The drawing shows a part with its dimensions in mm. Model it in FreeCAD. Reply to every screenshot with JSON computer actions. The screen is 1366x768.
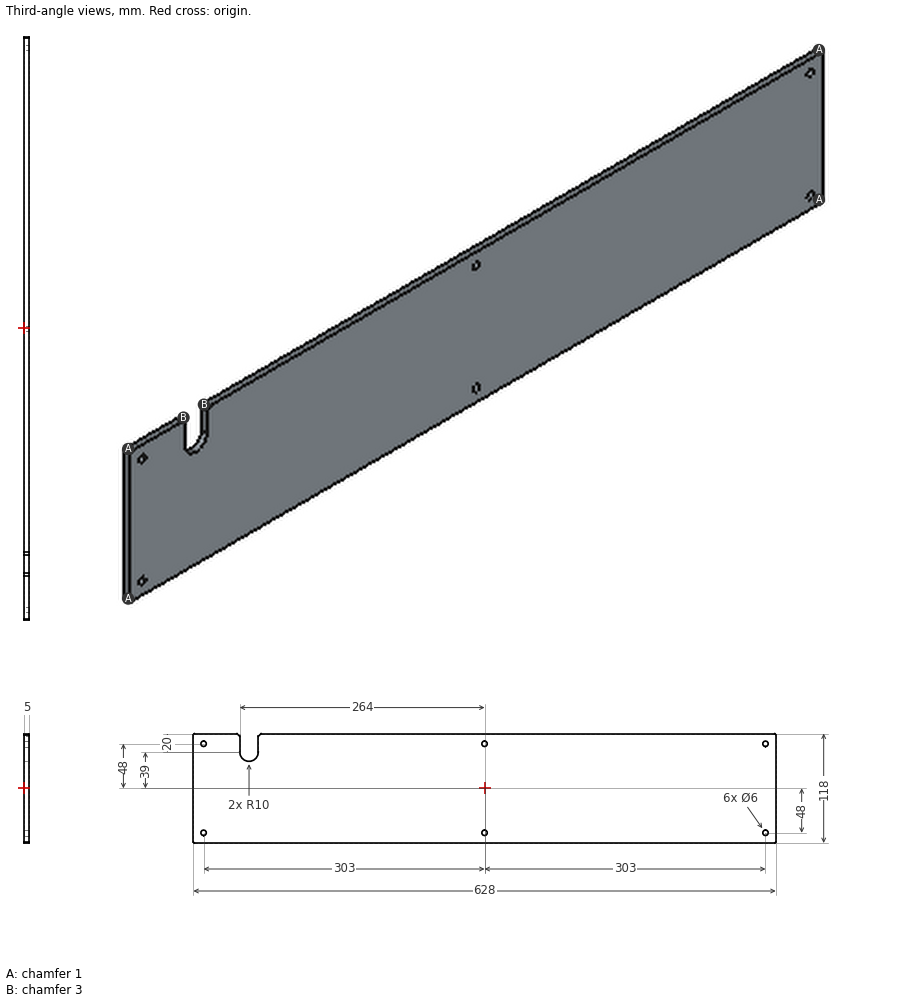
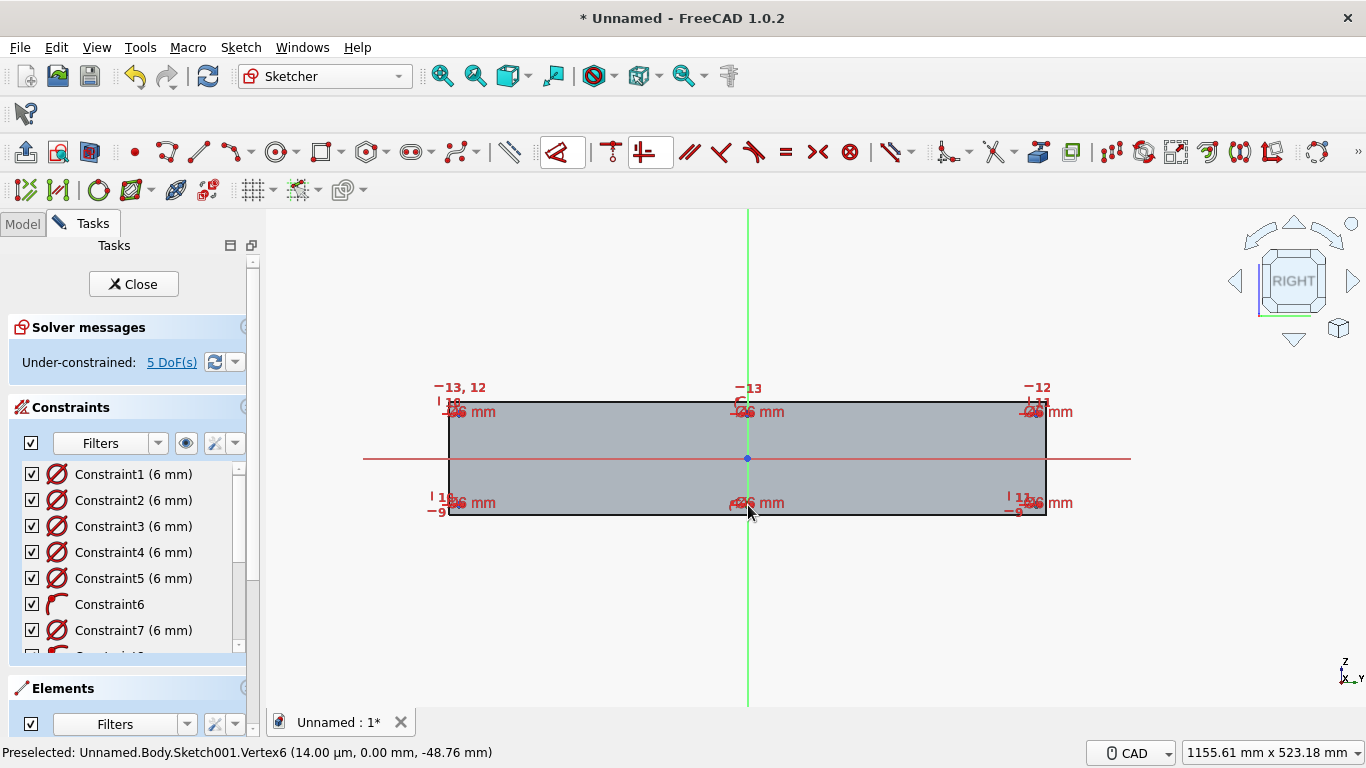
{"action": "key", "text": "h"}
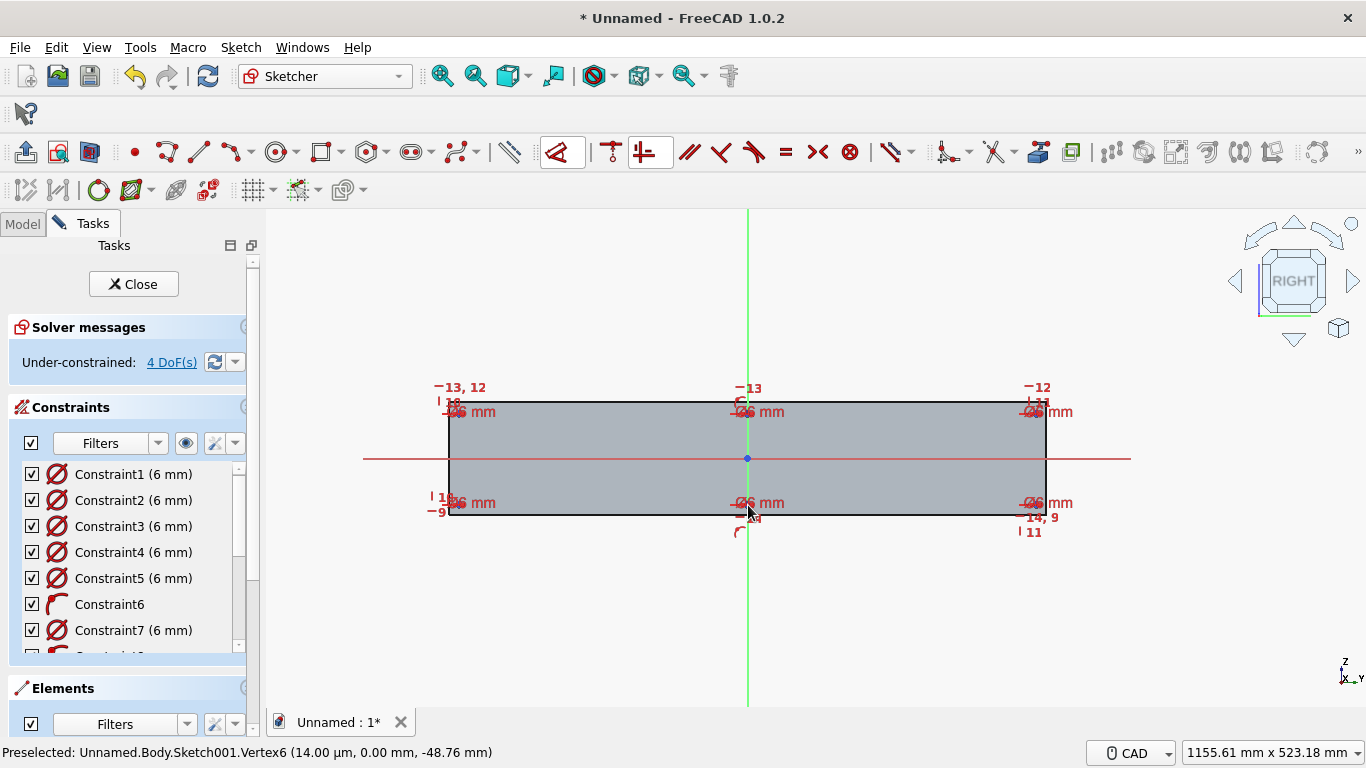
{"action": "left_click", "coordinate": [1036, 505]}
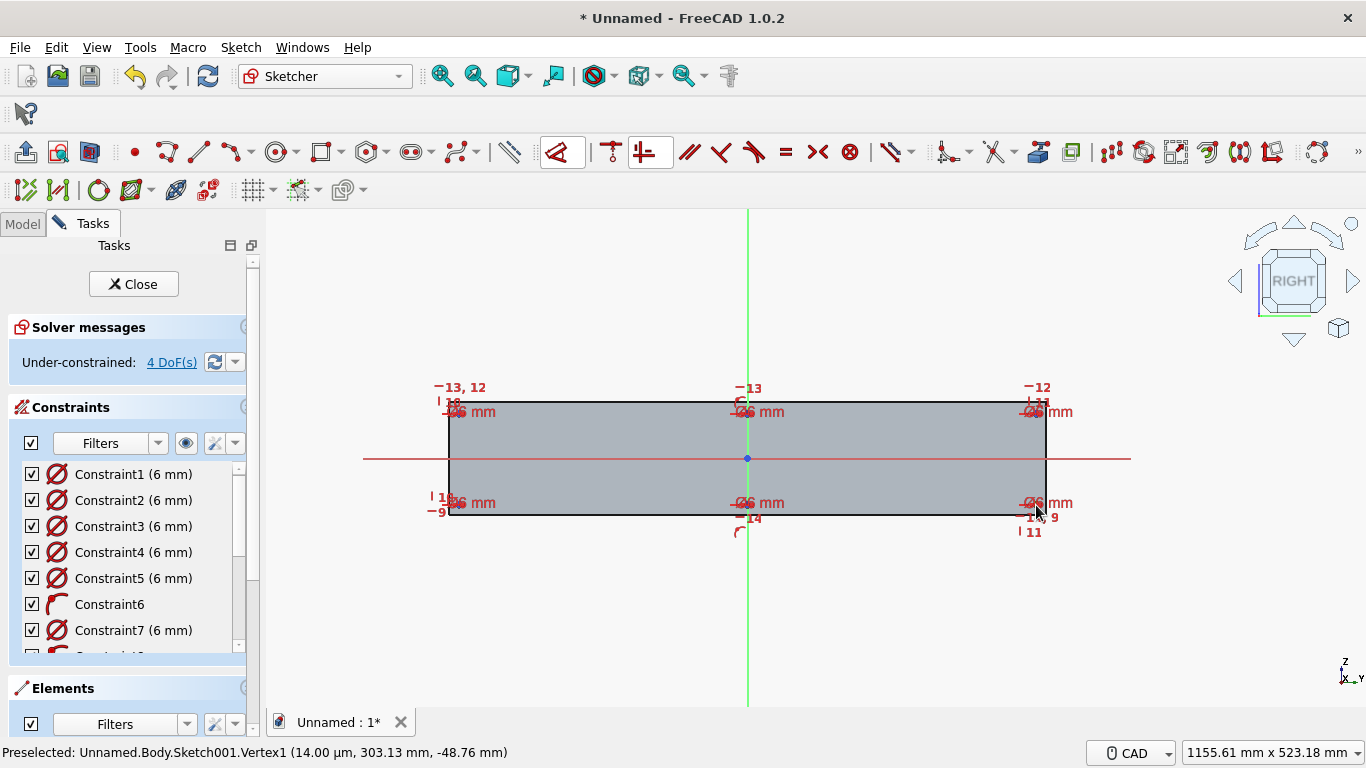
{"action": "left_click", "coordinate": [580, 152]}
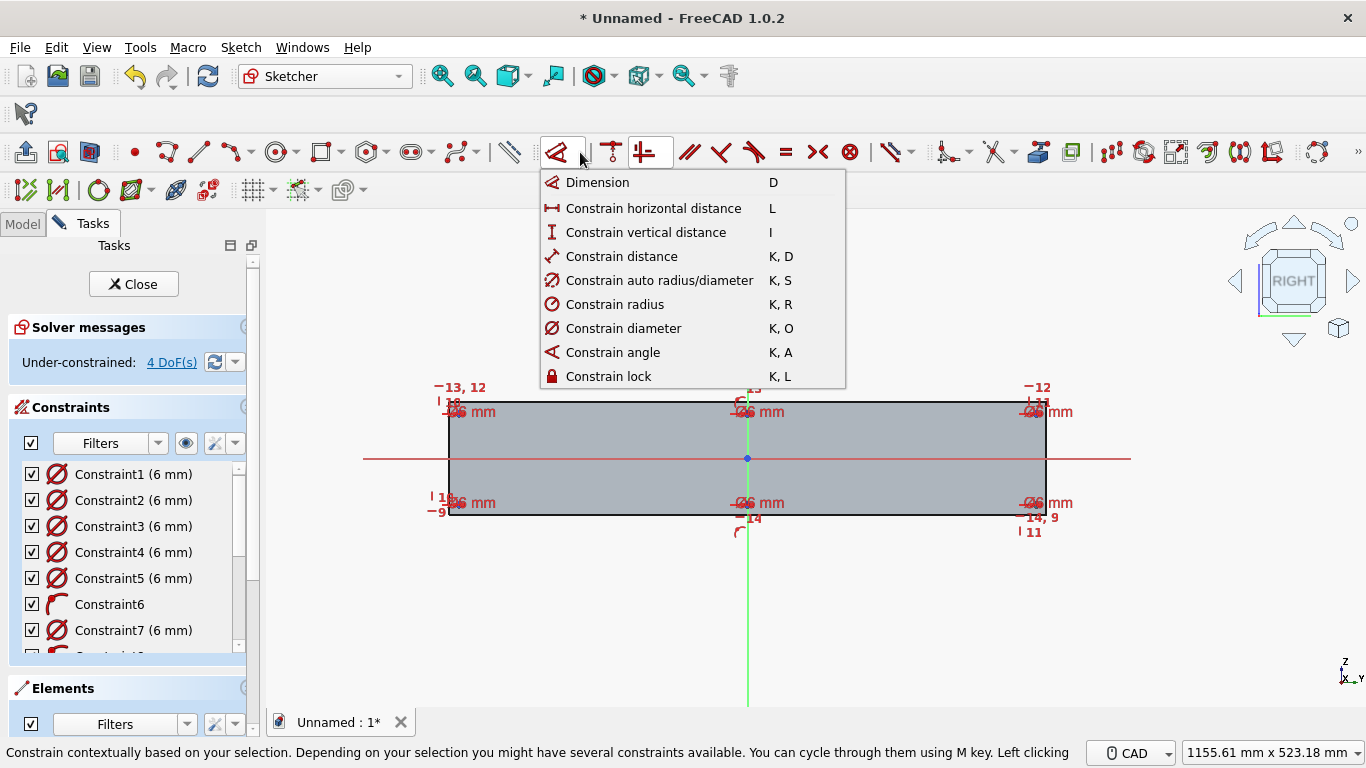
{"action": "left_click", "coordinate": [693, 232]}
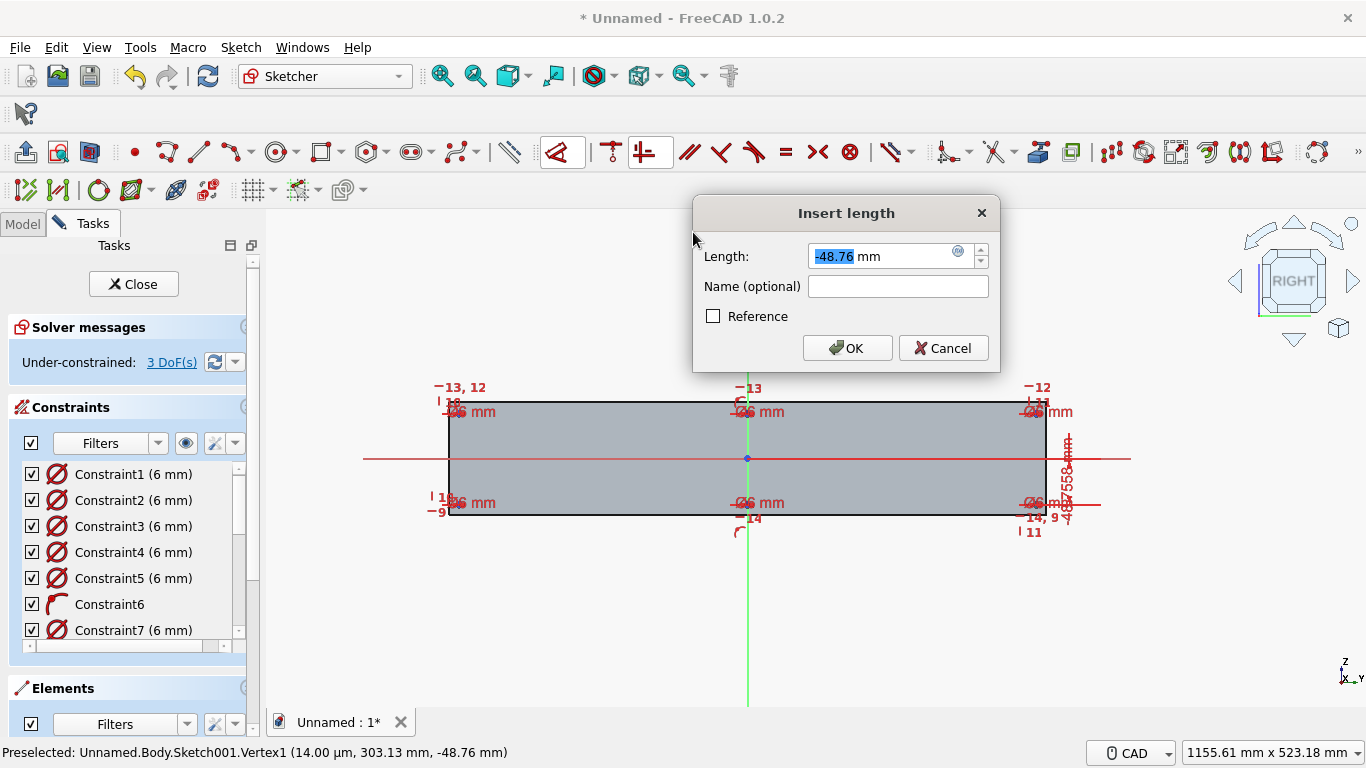
{"action": "type", "text": "-48"}
{"action": "key", "text": "Return"}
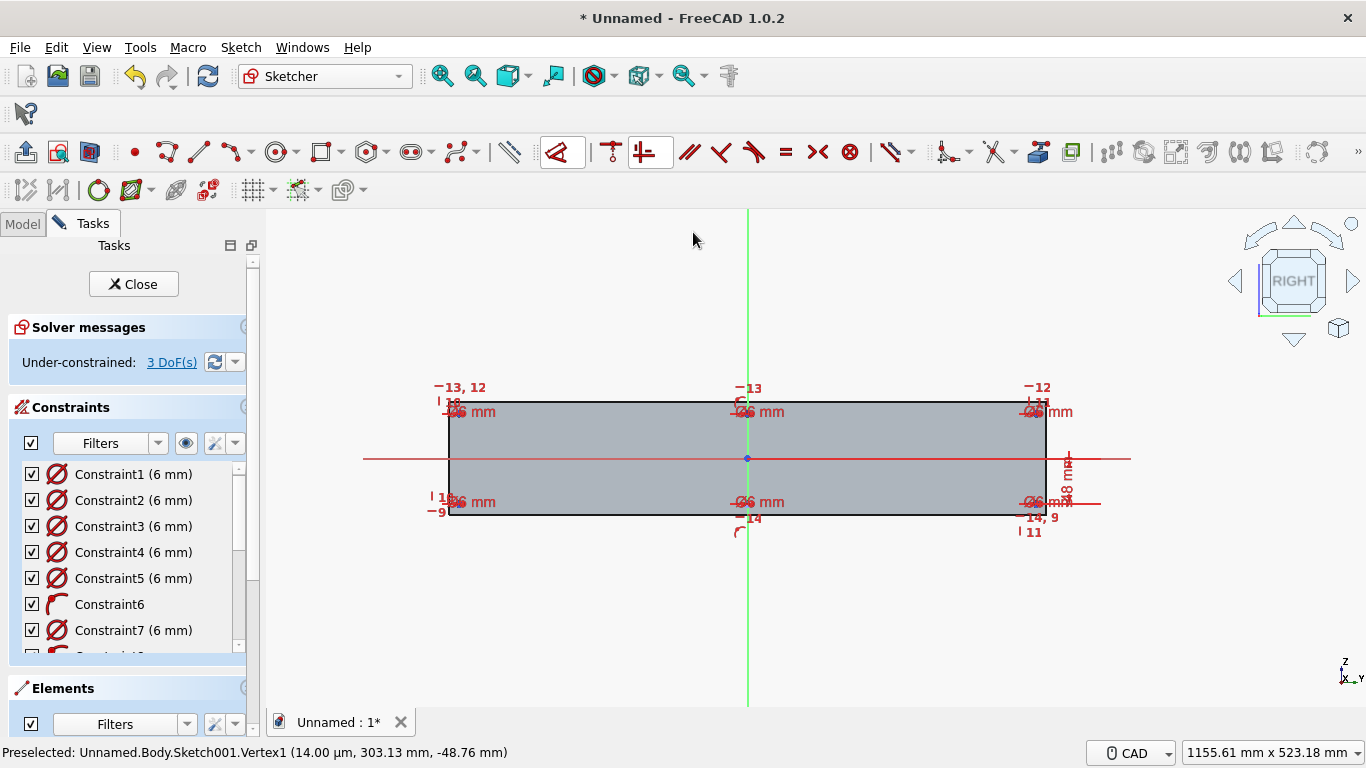
{"action": "left_click", "coordinate": [459, 414]}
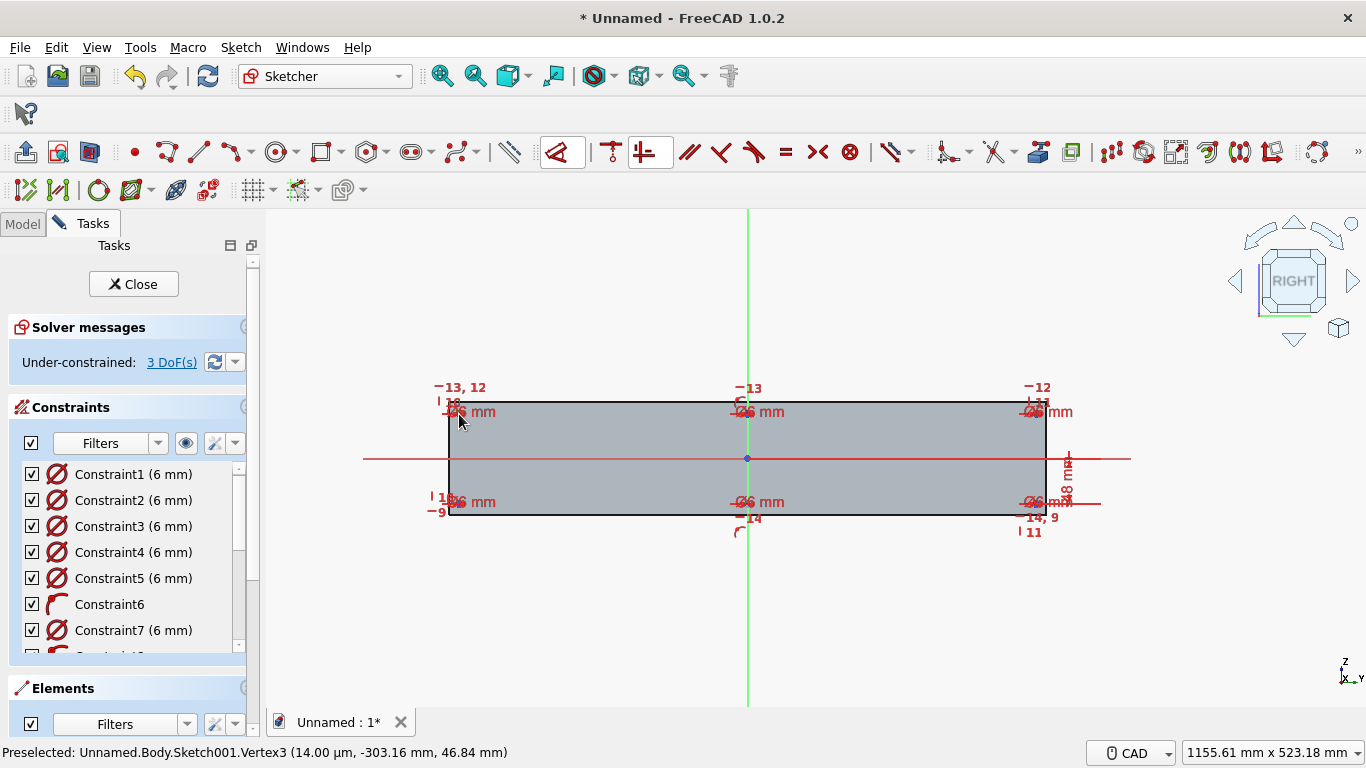
{"action": "key", "text": "i"}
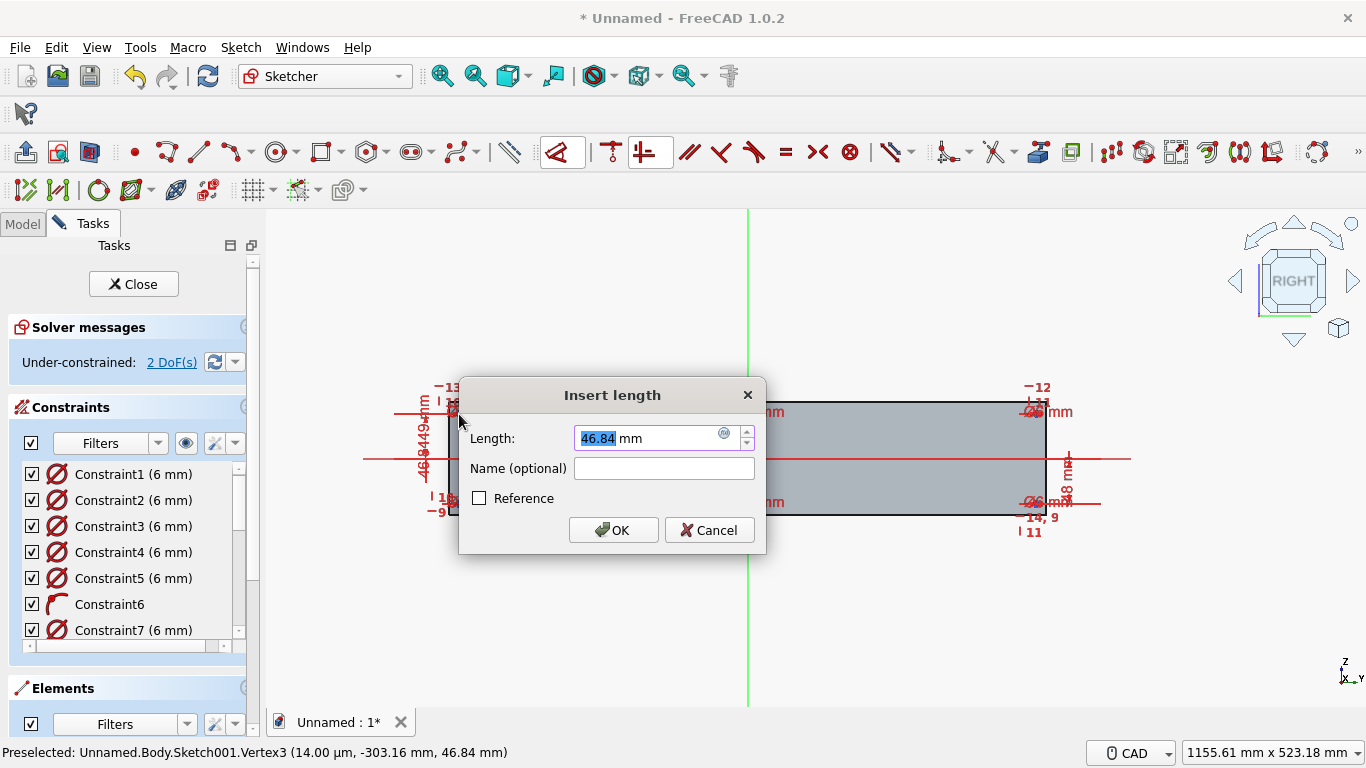
{"action": "type", "text": "48"}
{"action": "key", "text": "Return"}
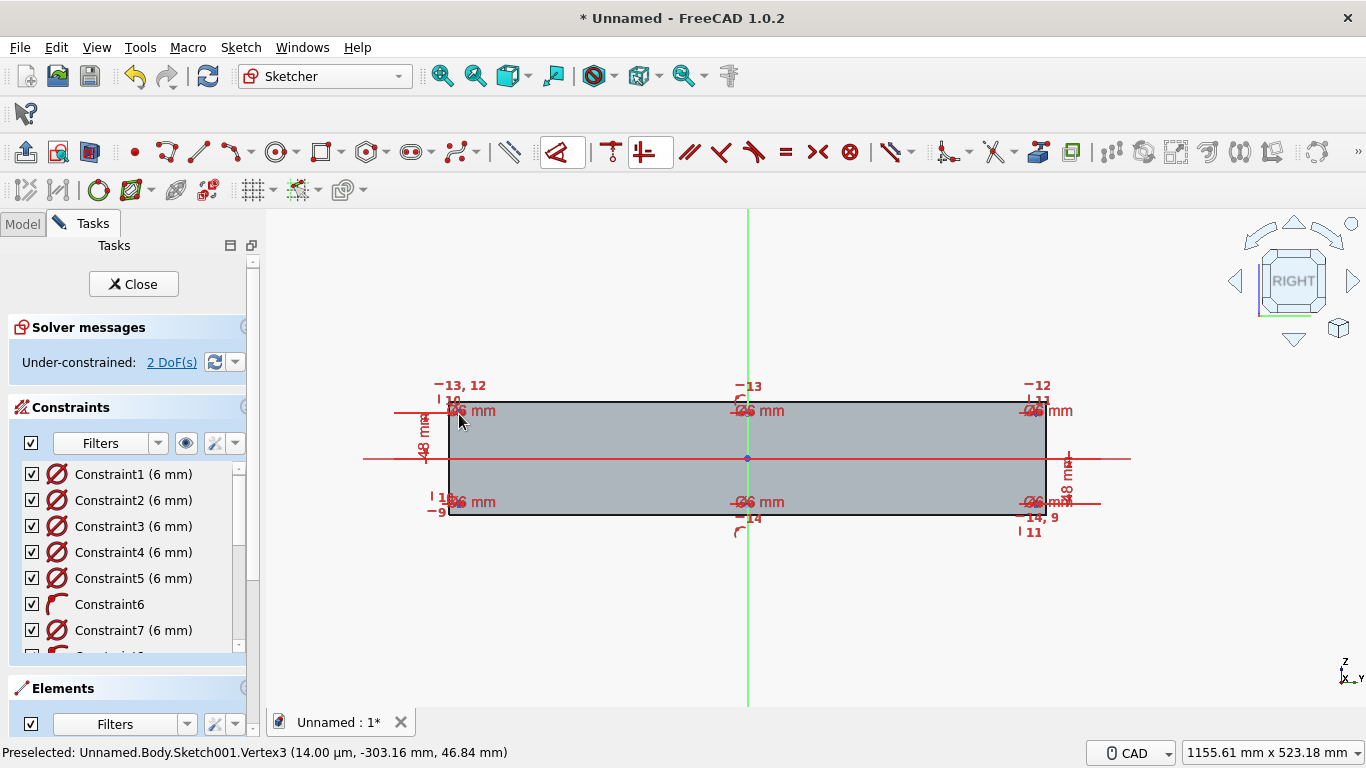
{"action": "left_click", "coordinate": [1036, 504]}